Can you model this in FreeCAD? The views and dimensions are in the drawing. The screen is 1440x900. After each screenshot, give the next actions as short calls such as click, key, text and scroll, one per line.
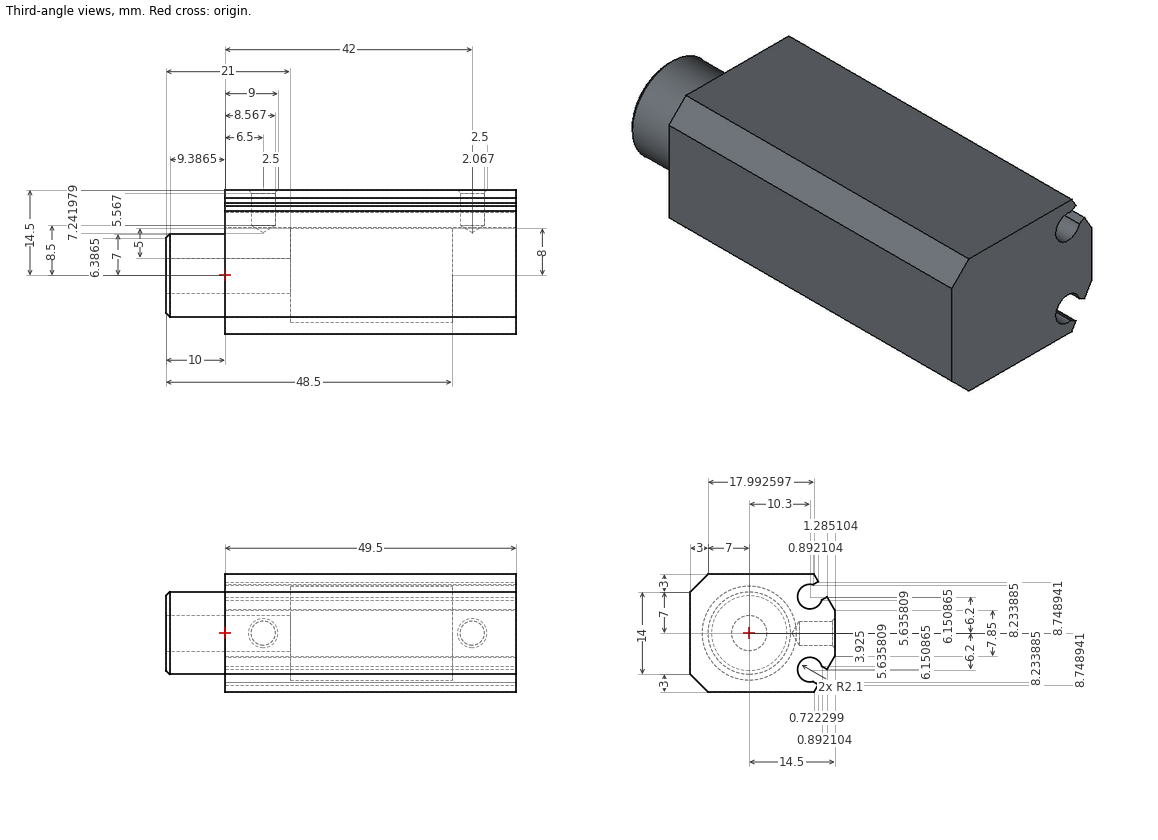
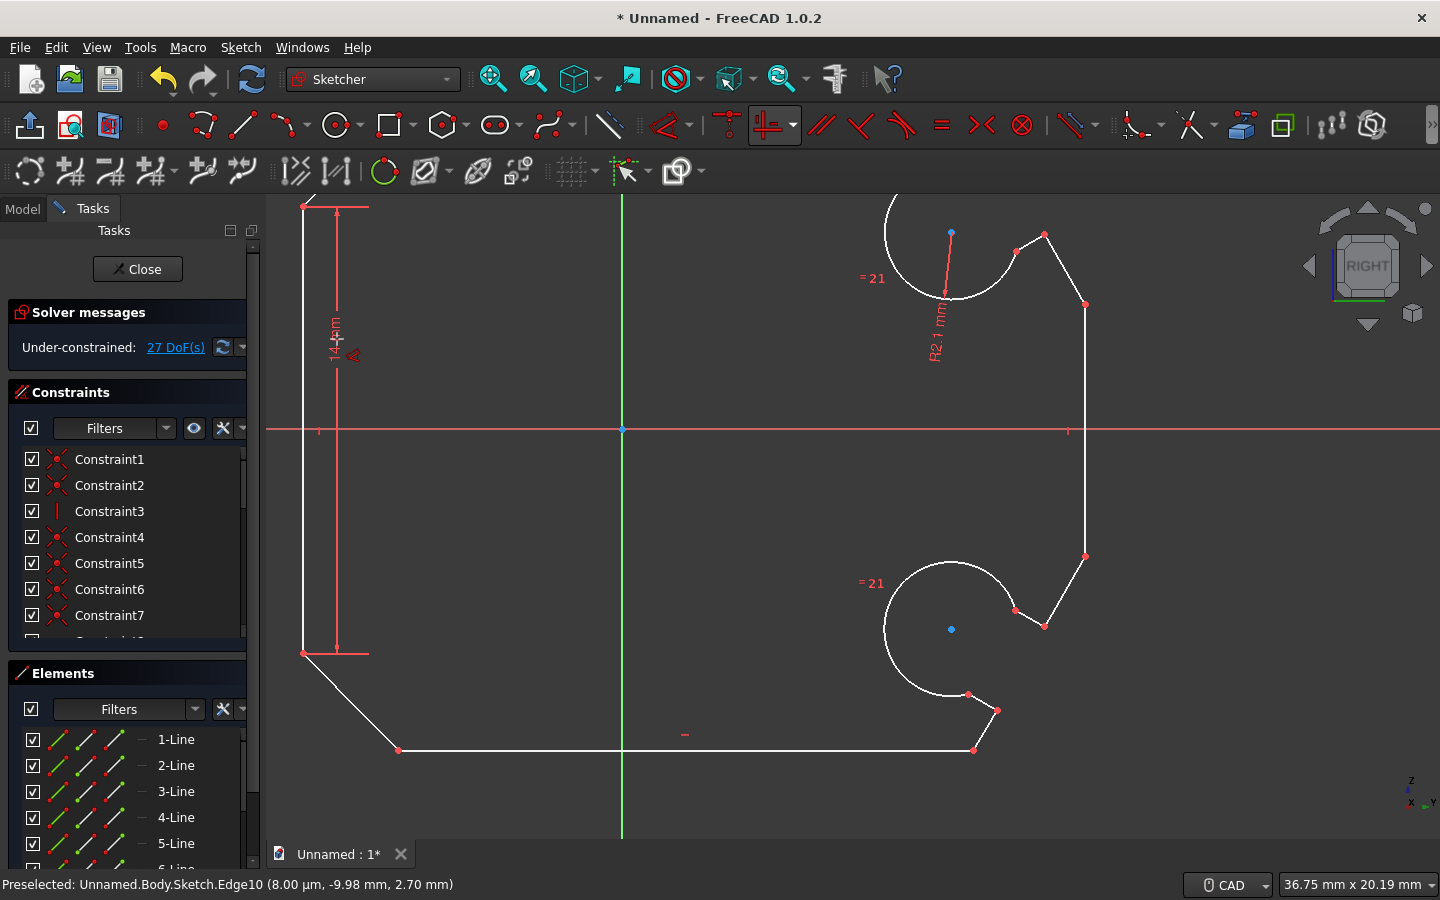
scroll(968, 694, down, 2)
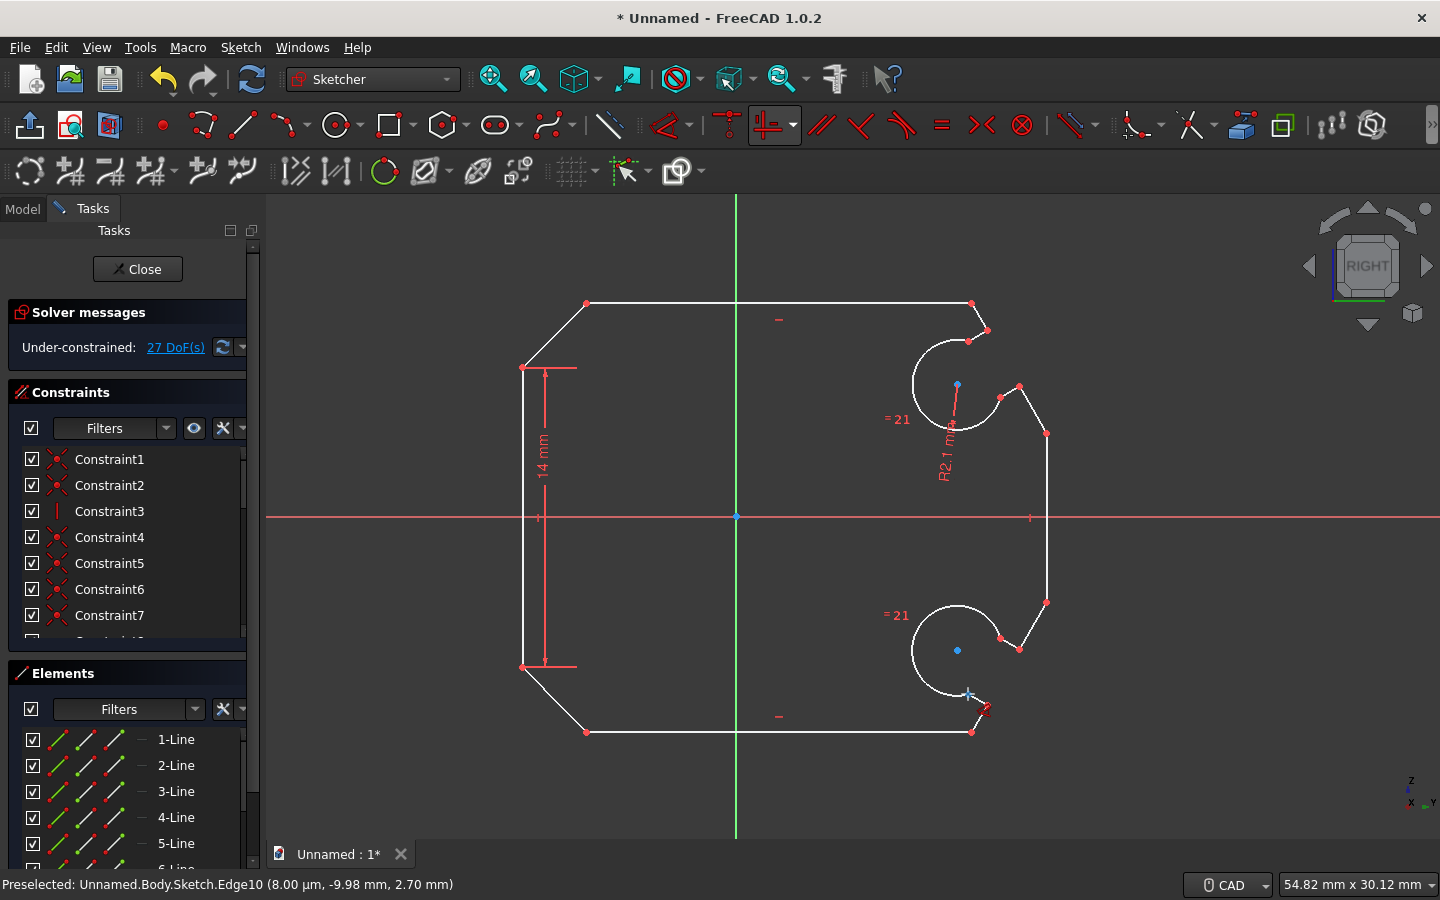
click(587, 303)
click(662, 269)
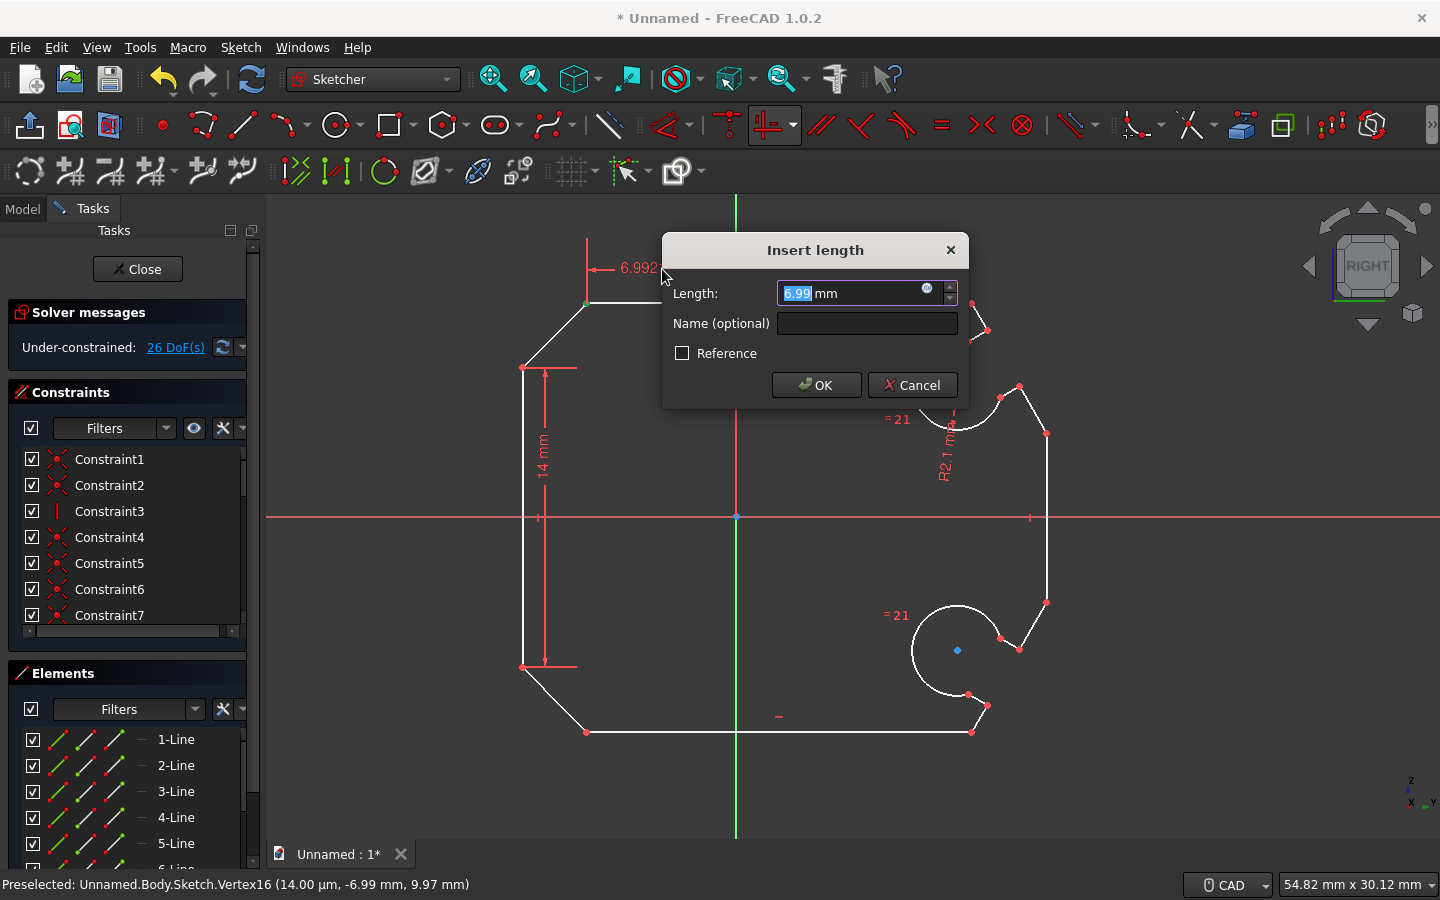
text(7)
key(Return)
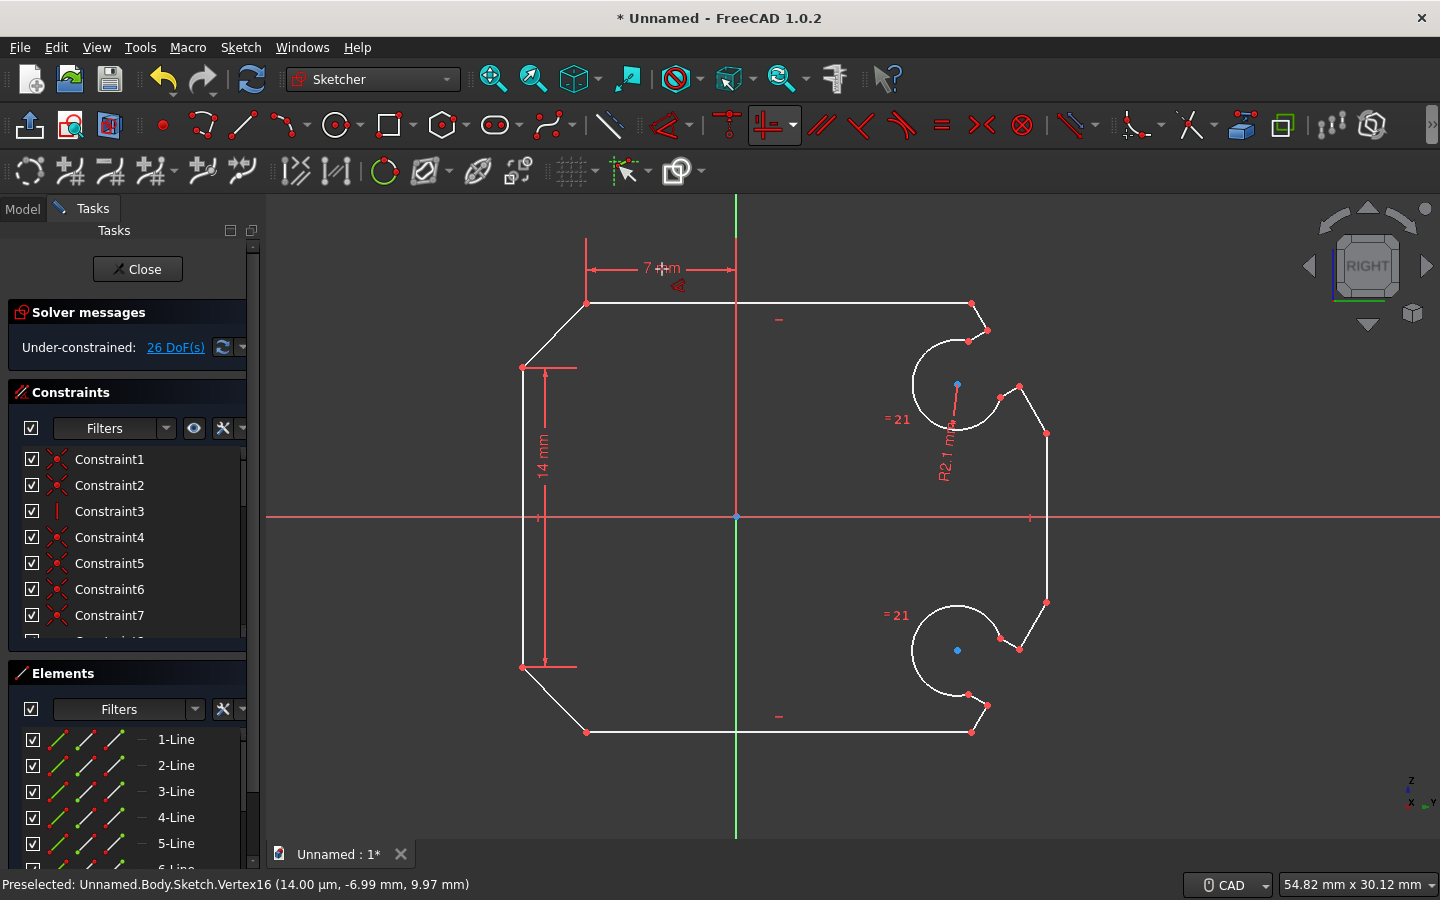
click(523, 368)
click(489, 408)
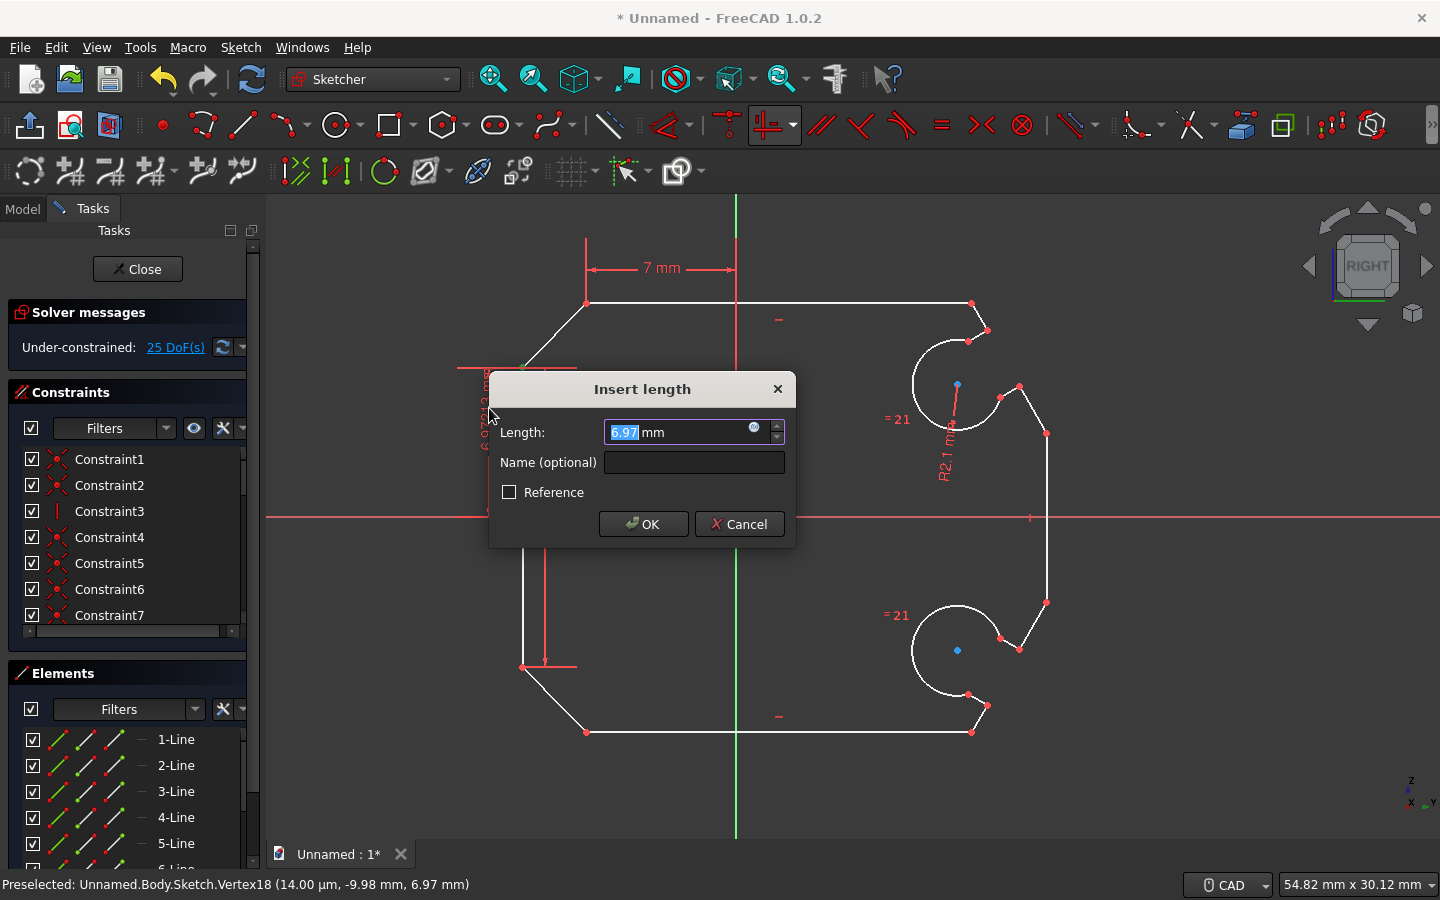
text(7)
key(Return)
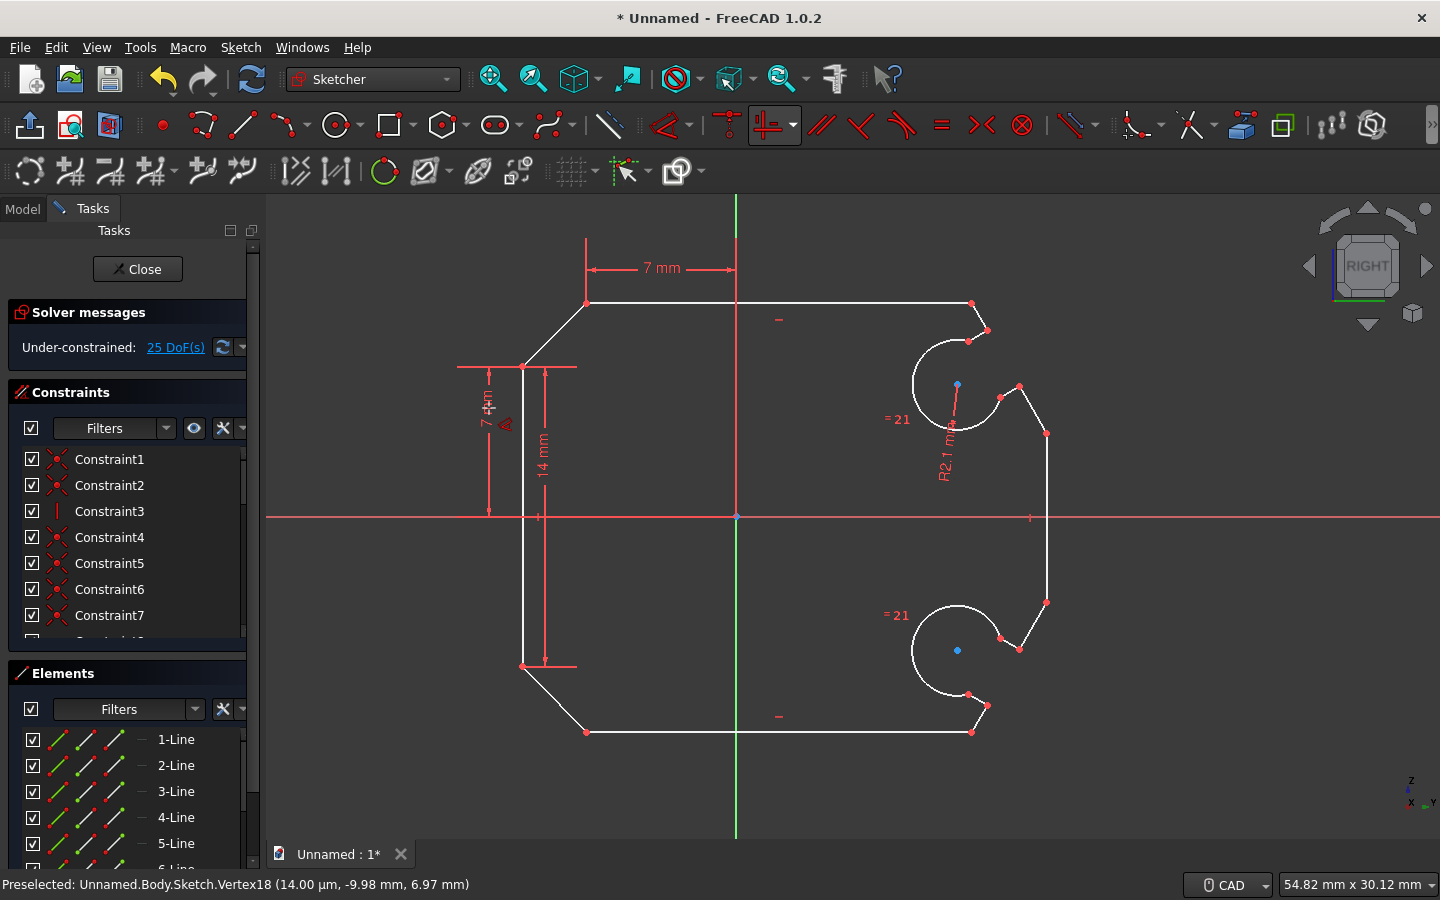
click(587, 732)
click(662, 766)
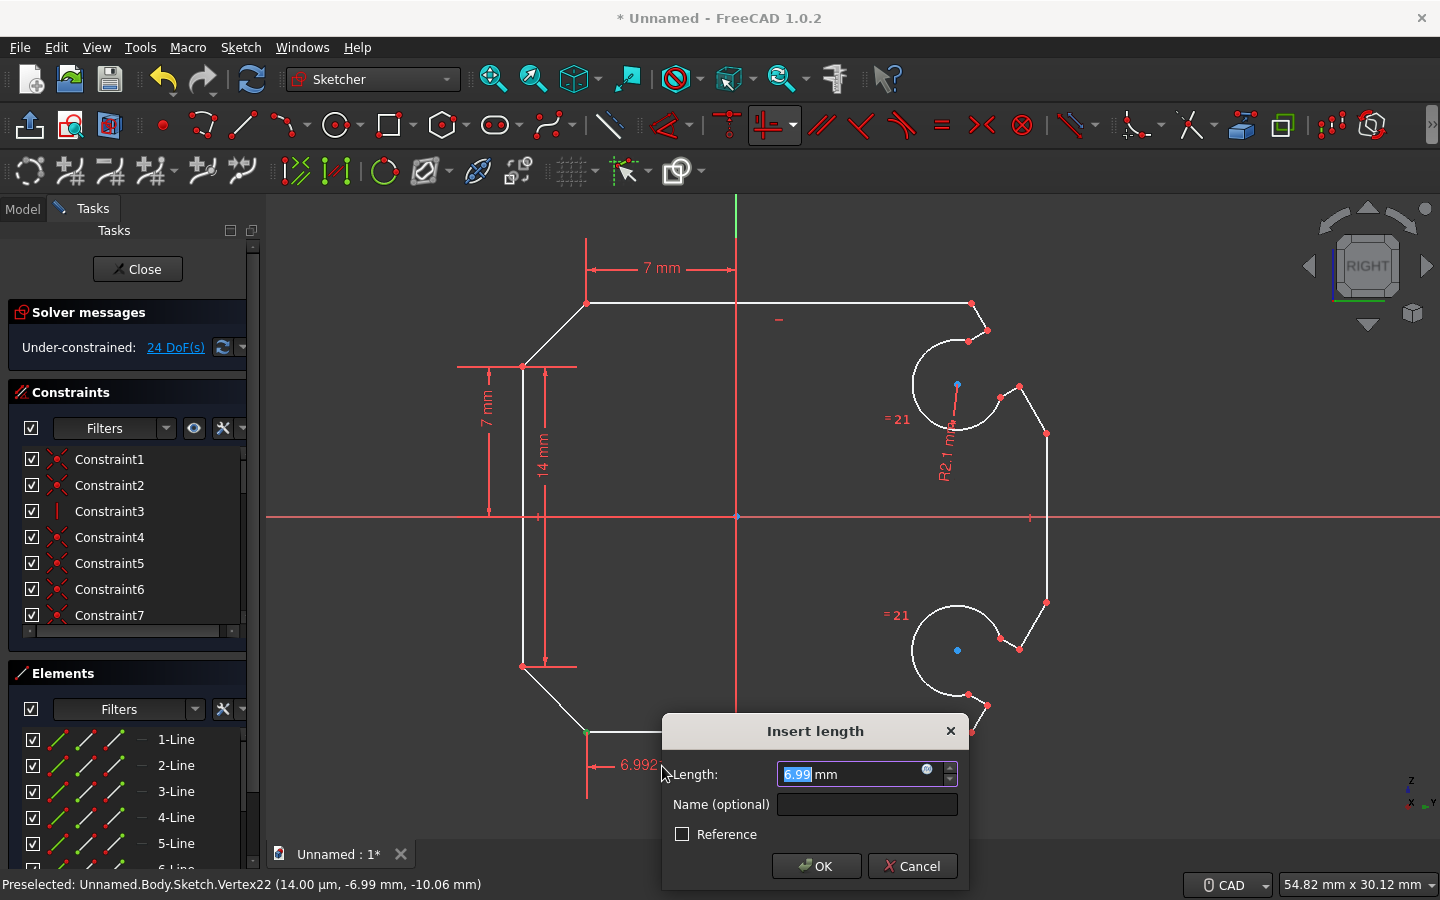
text(7)
key(Return)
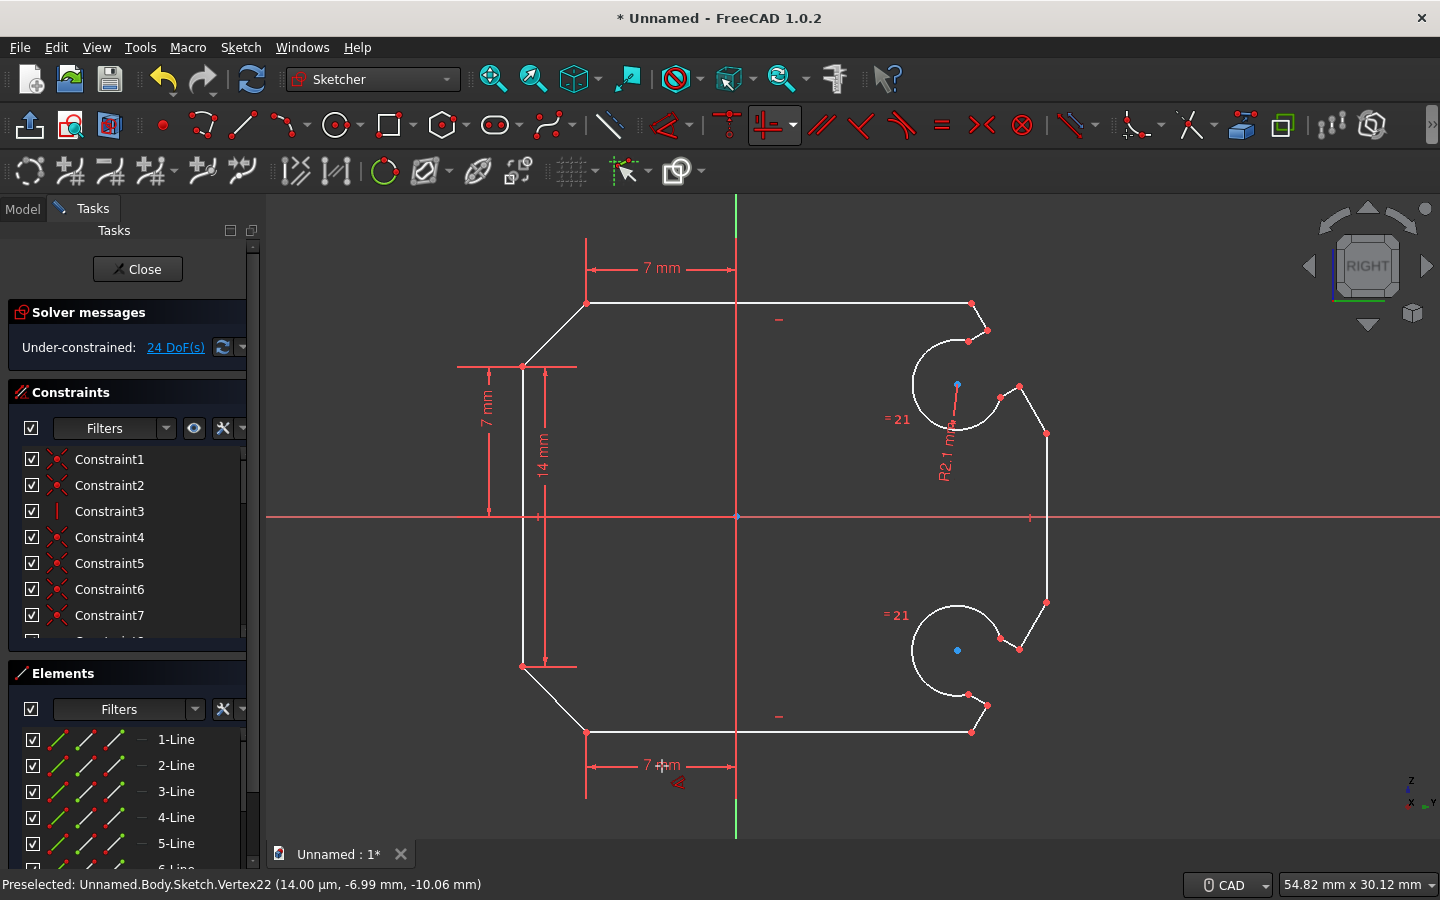
click(567, 322)
click(555, 269)